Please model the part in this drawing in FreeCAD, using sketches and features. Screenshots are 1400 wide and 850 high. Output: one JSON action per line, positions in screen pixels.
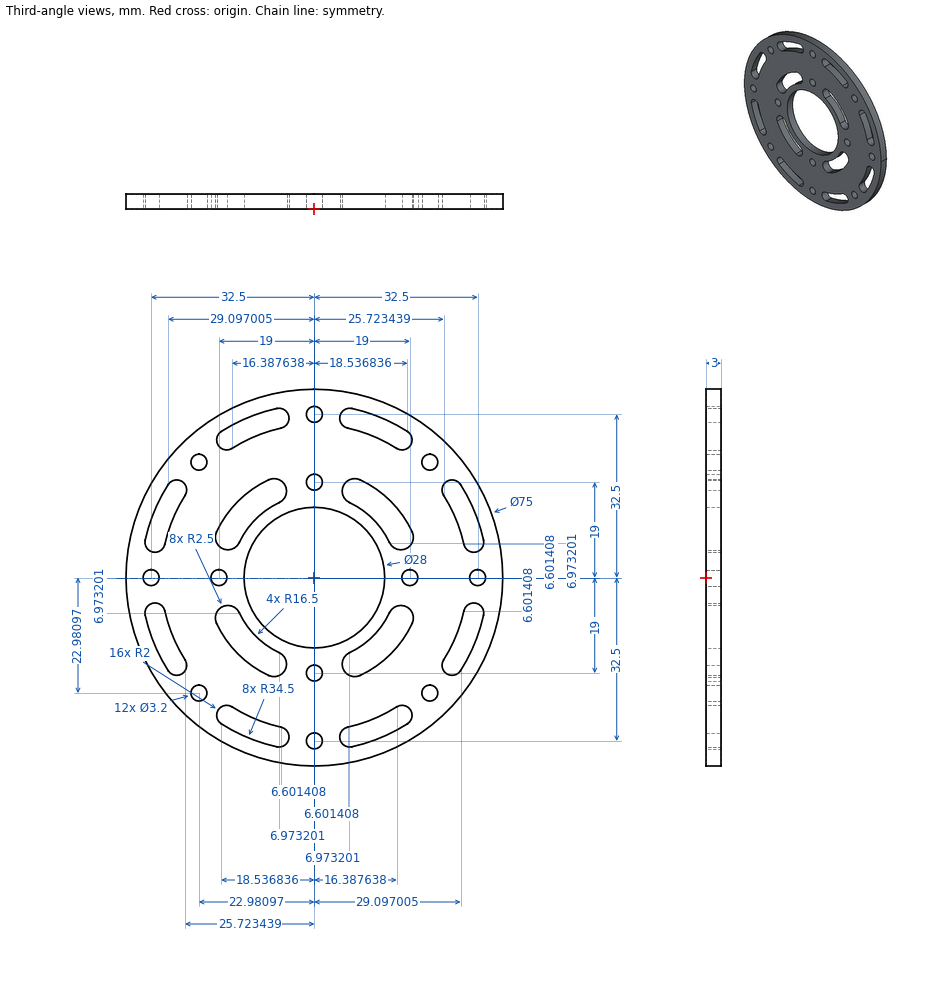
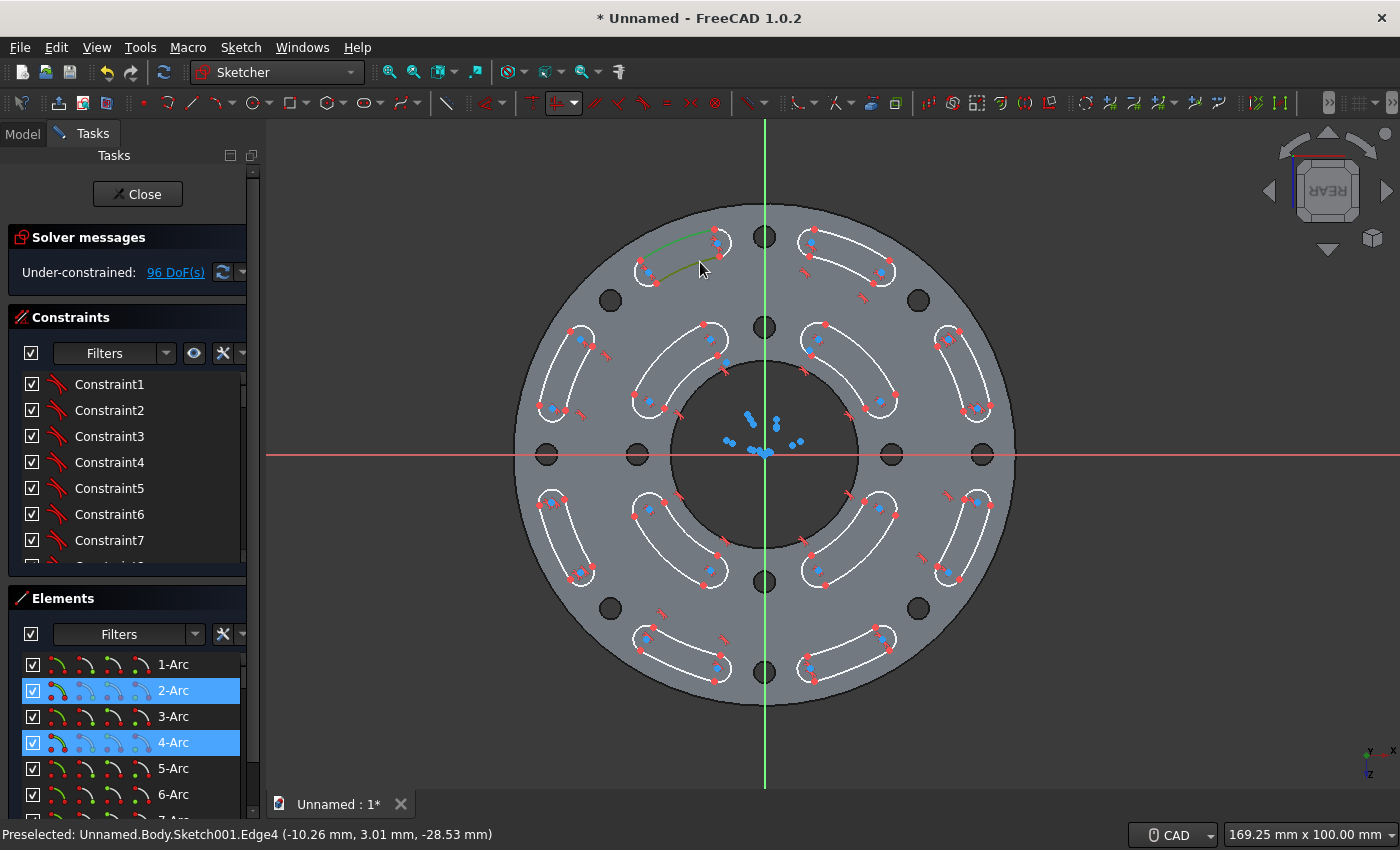
{"action": "left_click", "coordinate": [532, 104]}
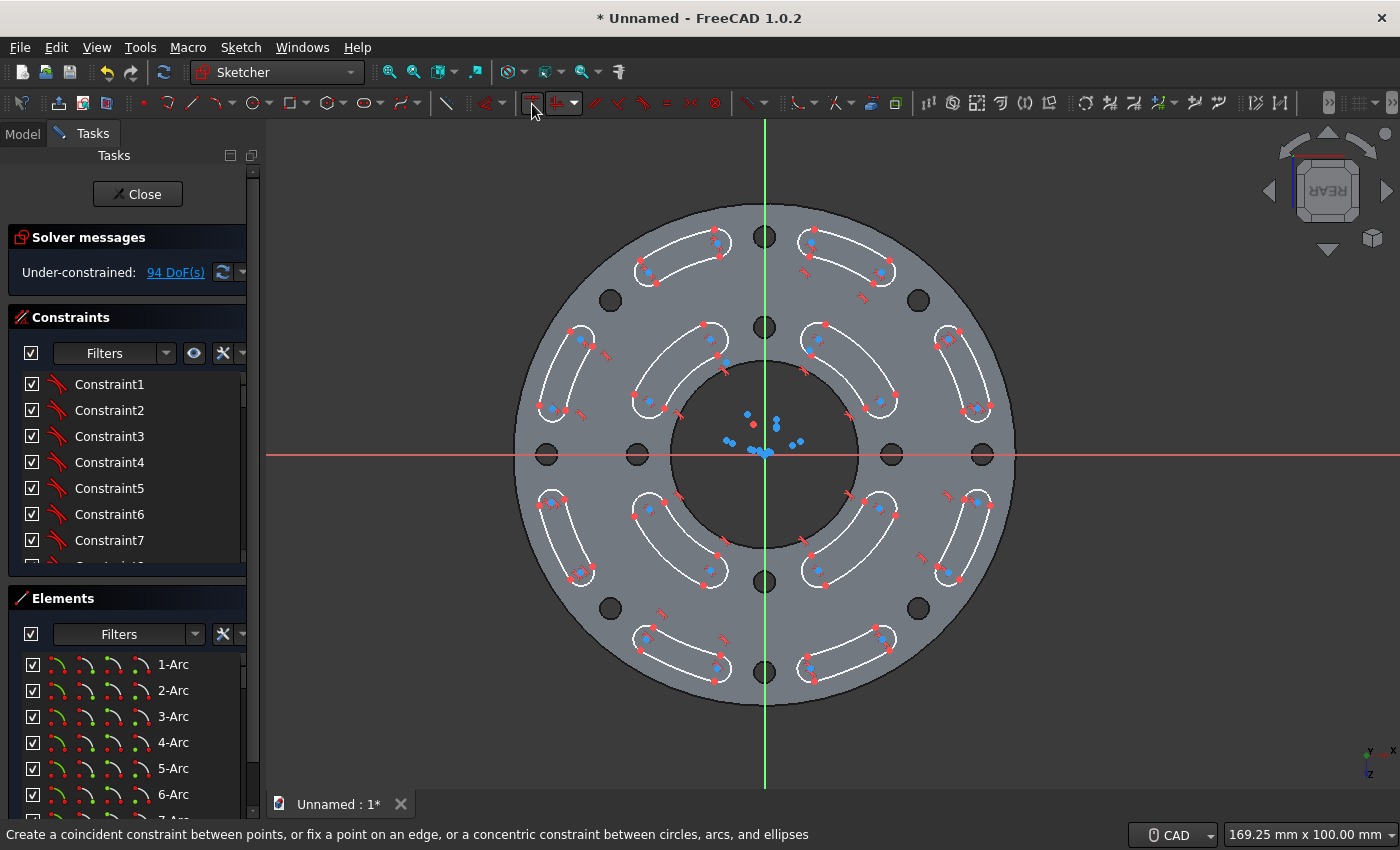
{"action": "left_click", "coordinate": [691, 236]}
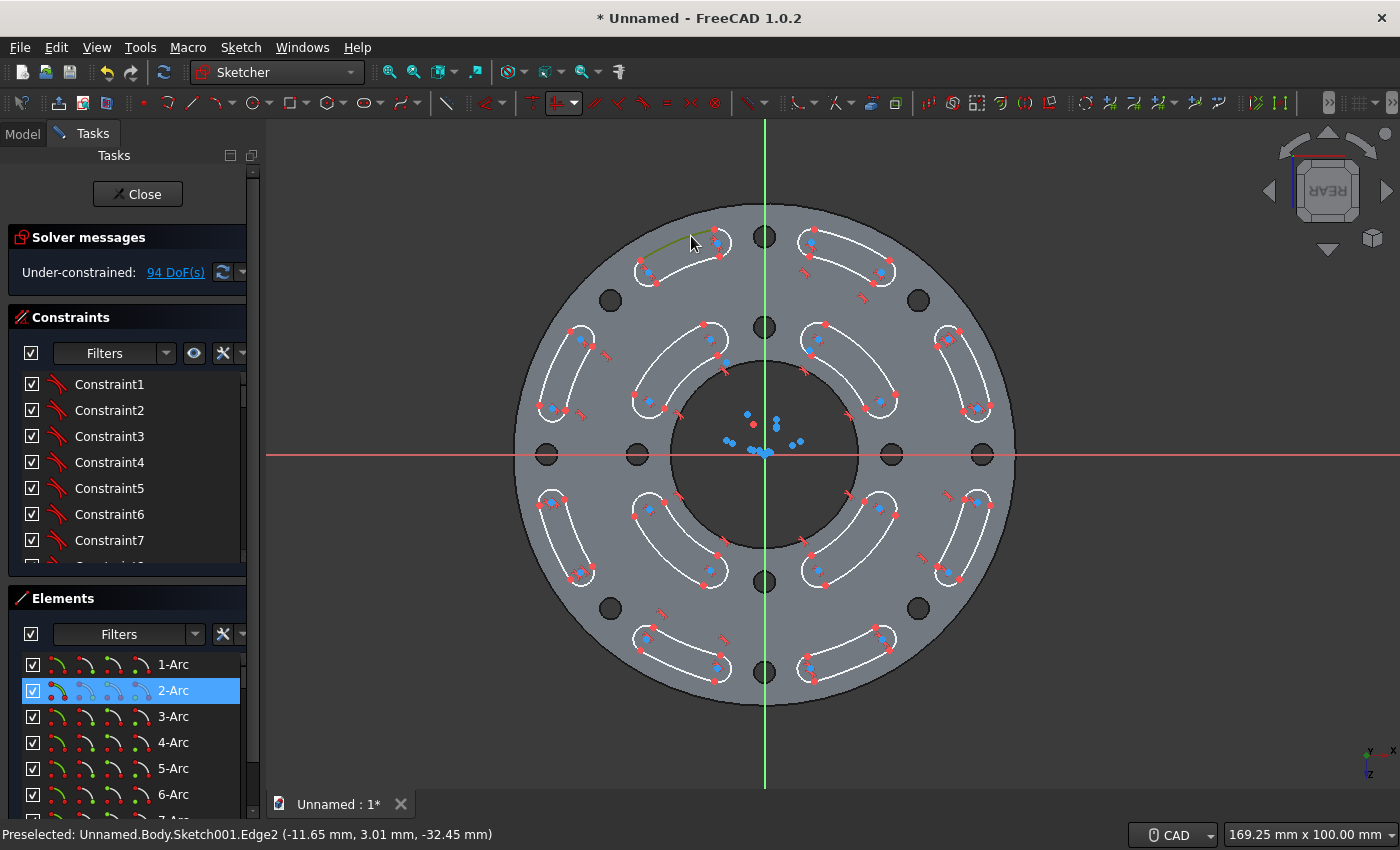
{"action": "left_click", "coordinate": [698, 367]}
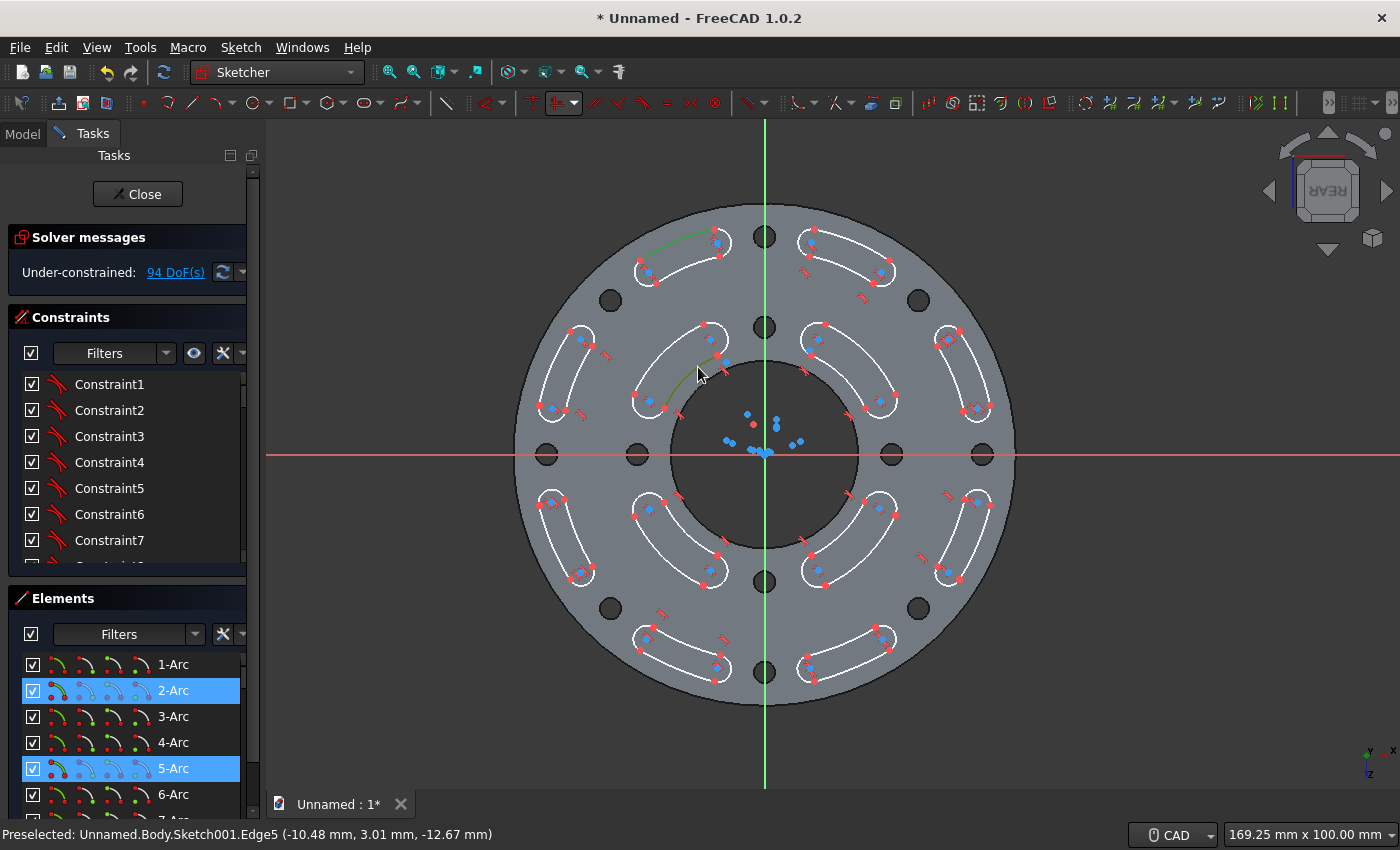
{"action": "left_click", "coordinate": [532, 104]}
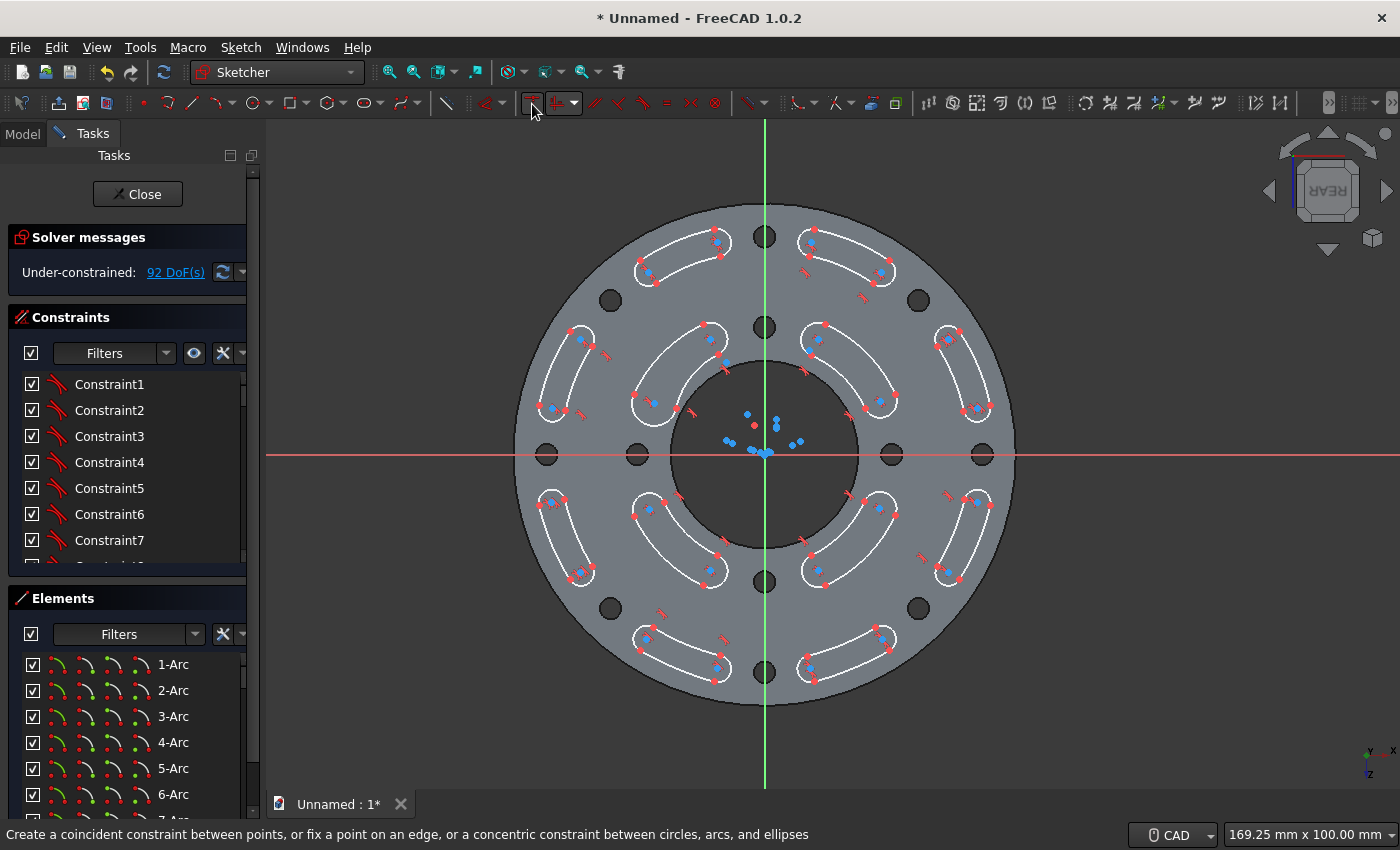
{"action": "left_click", "coordinate": [691, 236]}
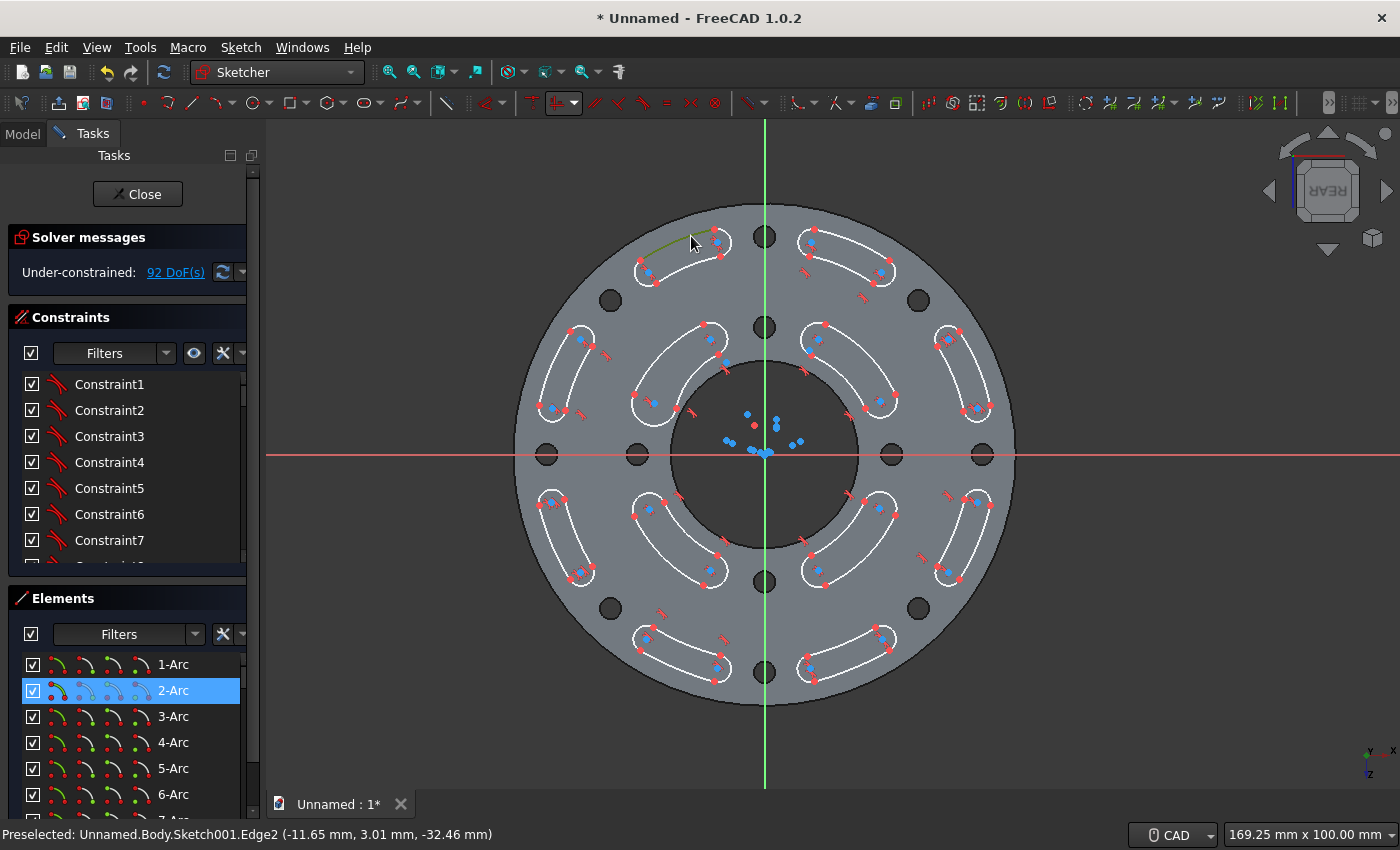
{"action": "left_click", "coordinate": [678, 340]}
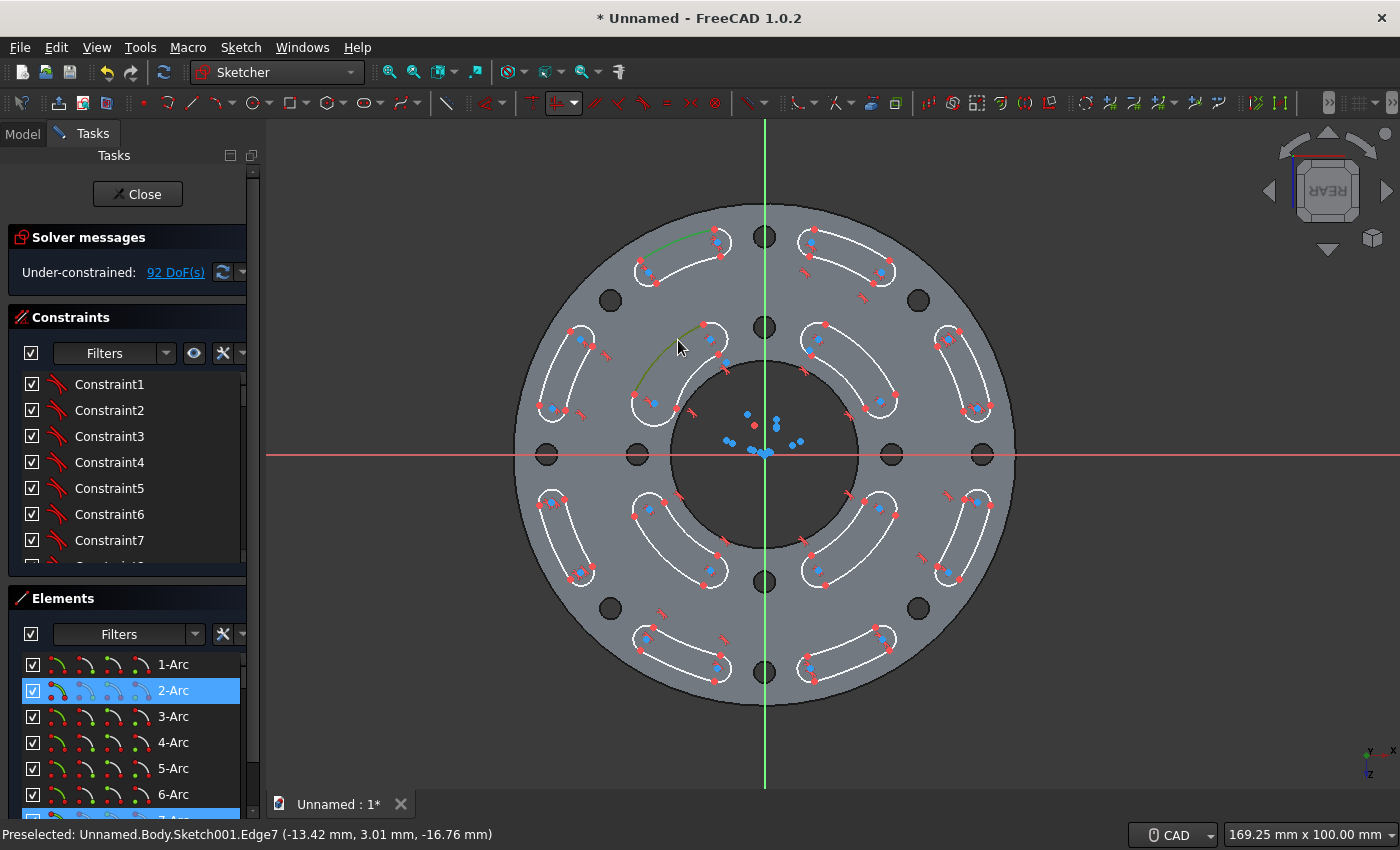
{"action": "left_click", "coordinate": [532, 104]}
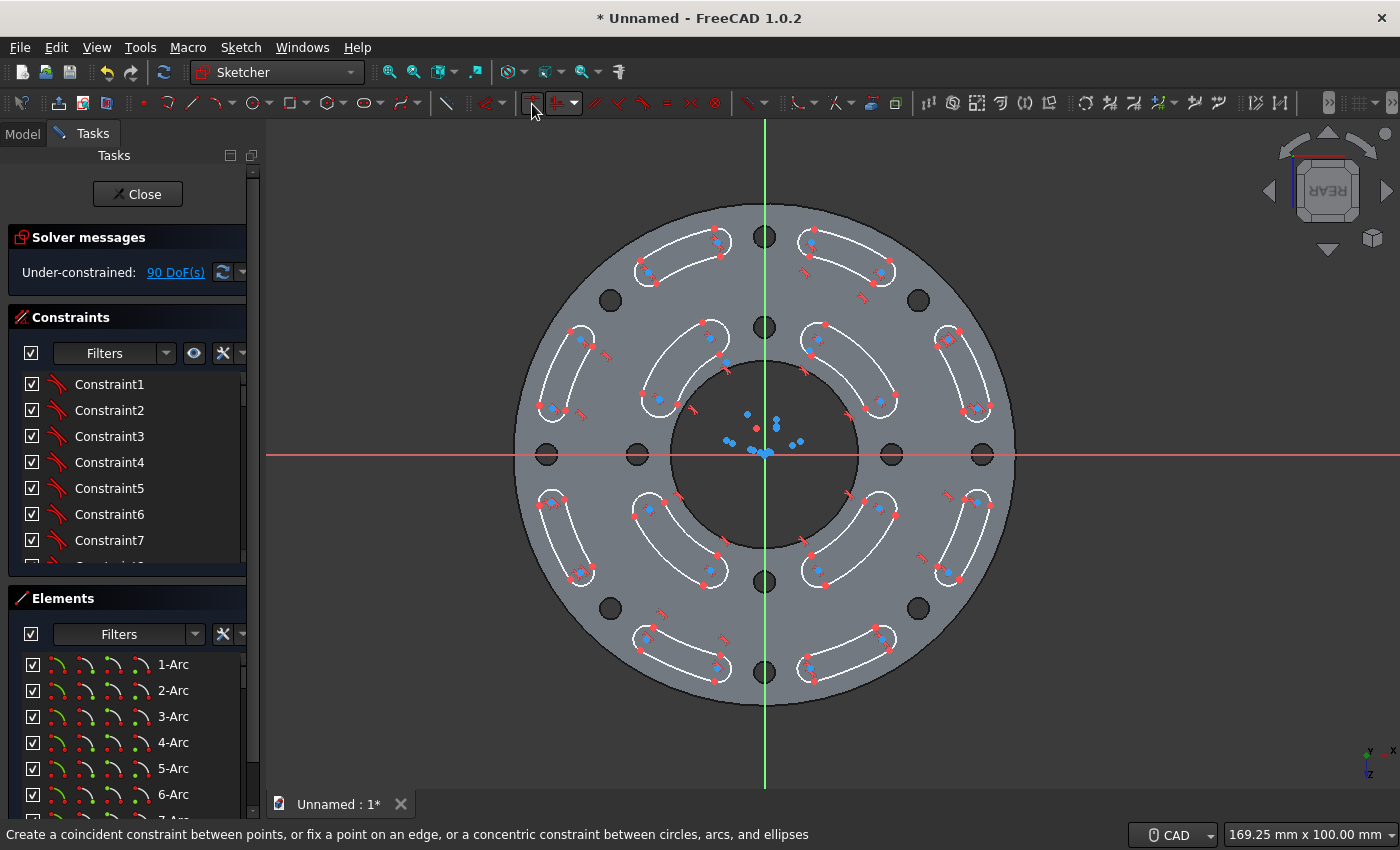
{"action": "left_click", "coordinate": [691, 235]}